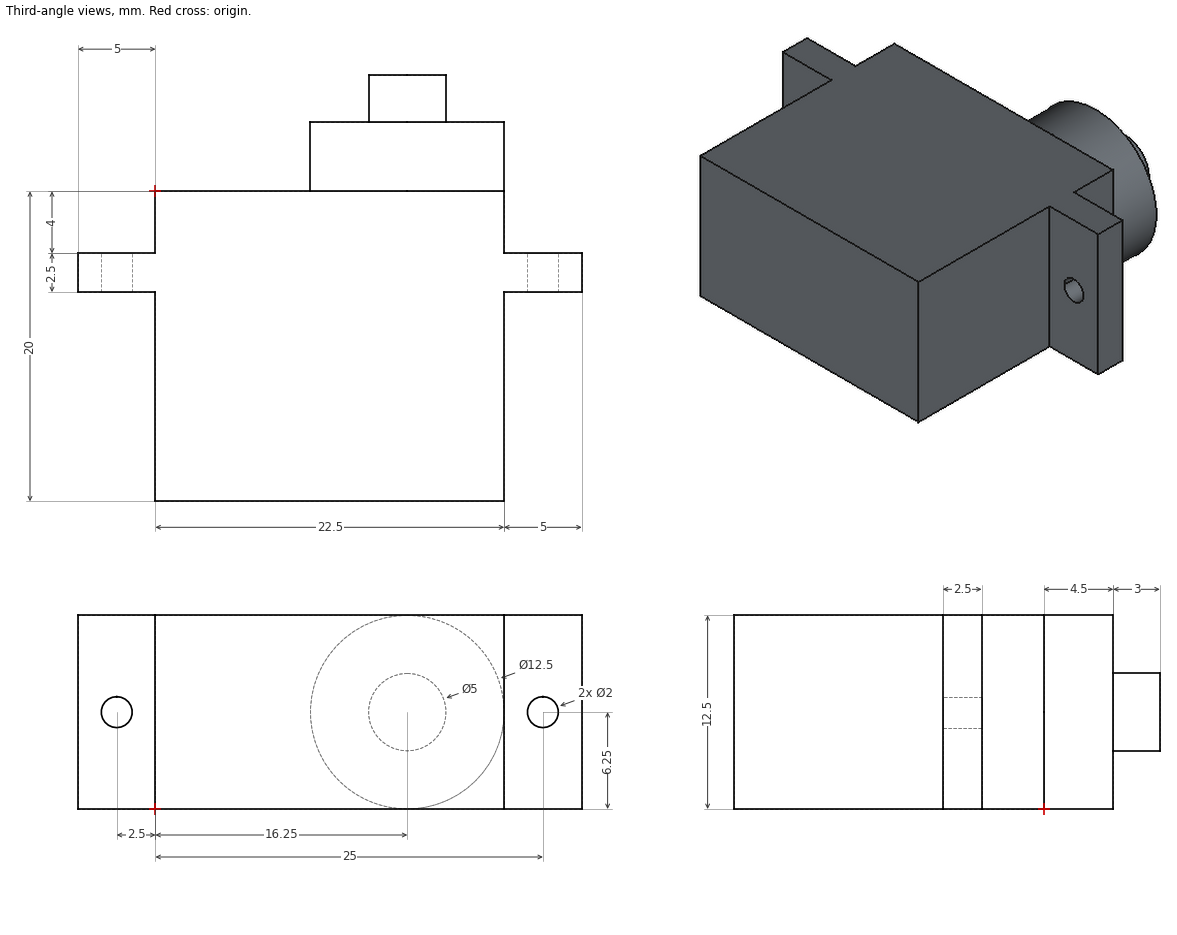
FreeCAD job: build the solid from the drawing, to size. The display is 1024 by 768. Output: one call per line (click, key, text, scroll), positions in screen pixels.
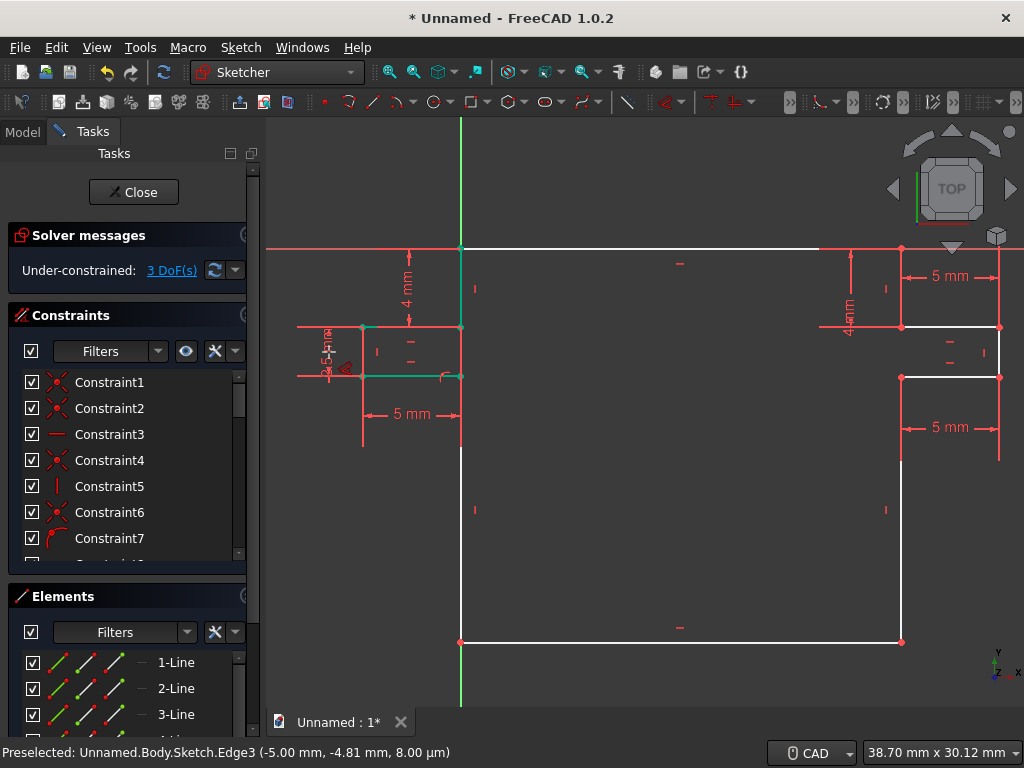
scroll(364, 345, down, 2)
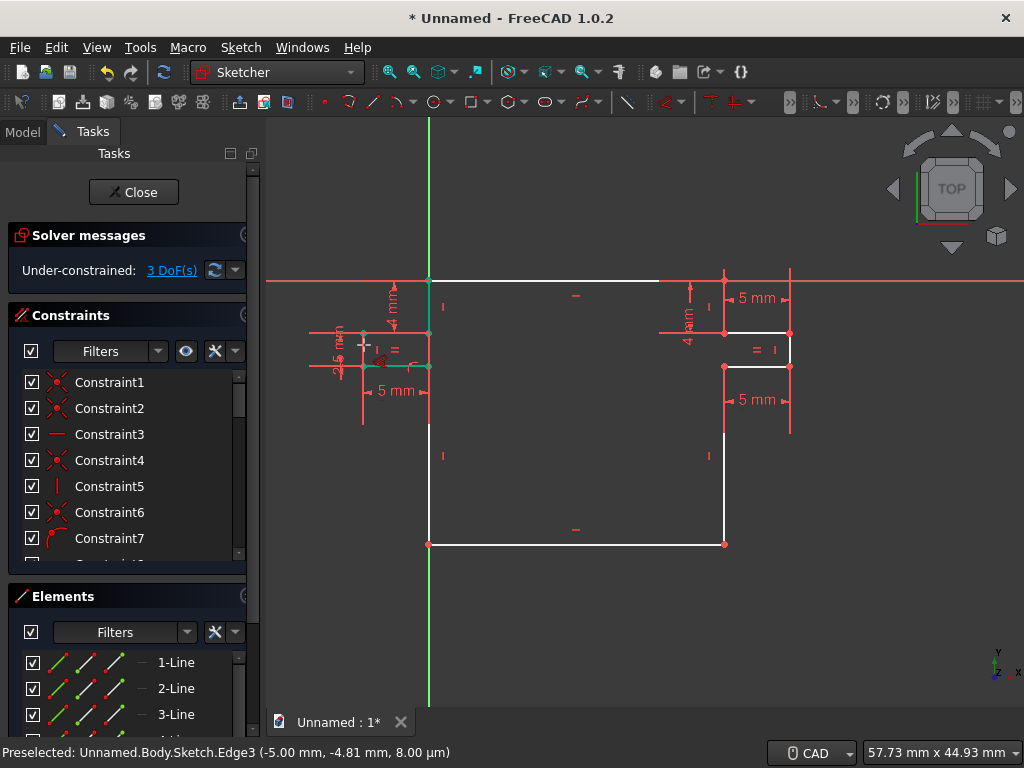
scroll(790, 357, up, 2)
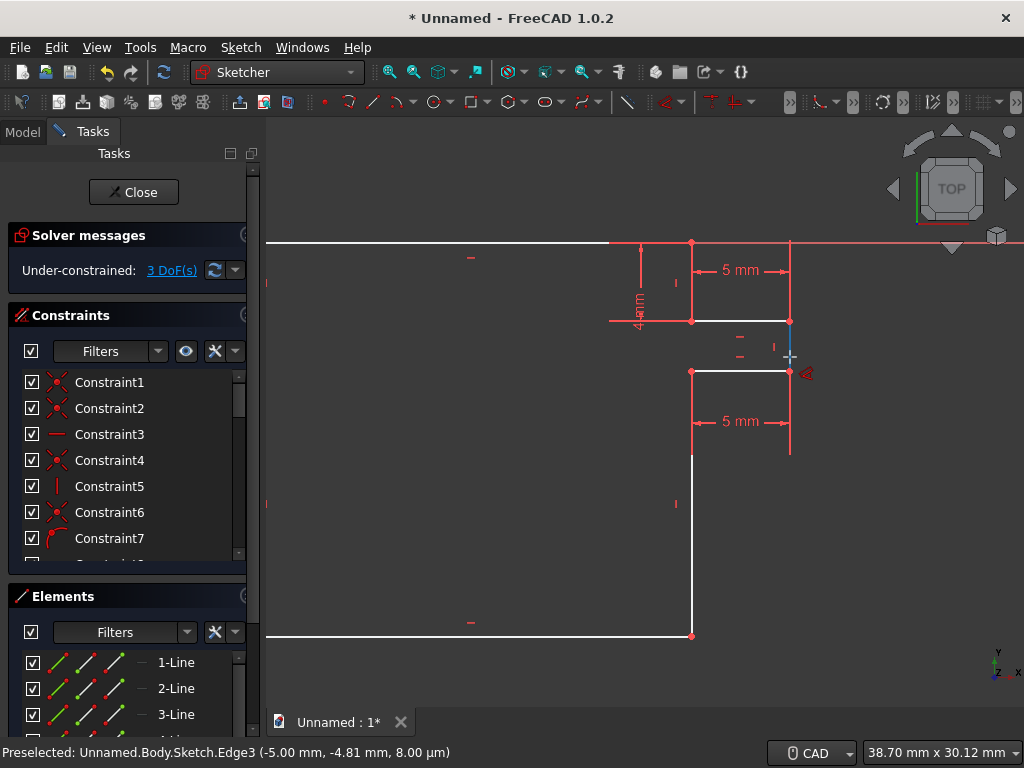
click(790, 356)
click(824, 346)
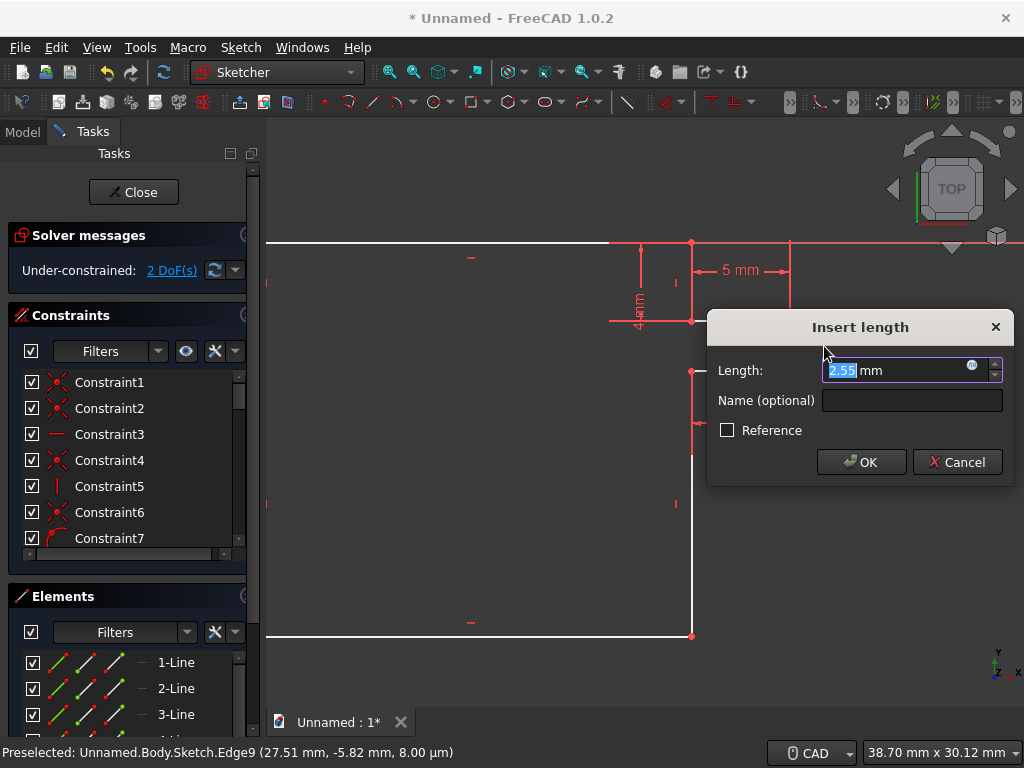
text(2.5)
key(Return)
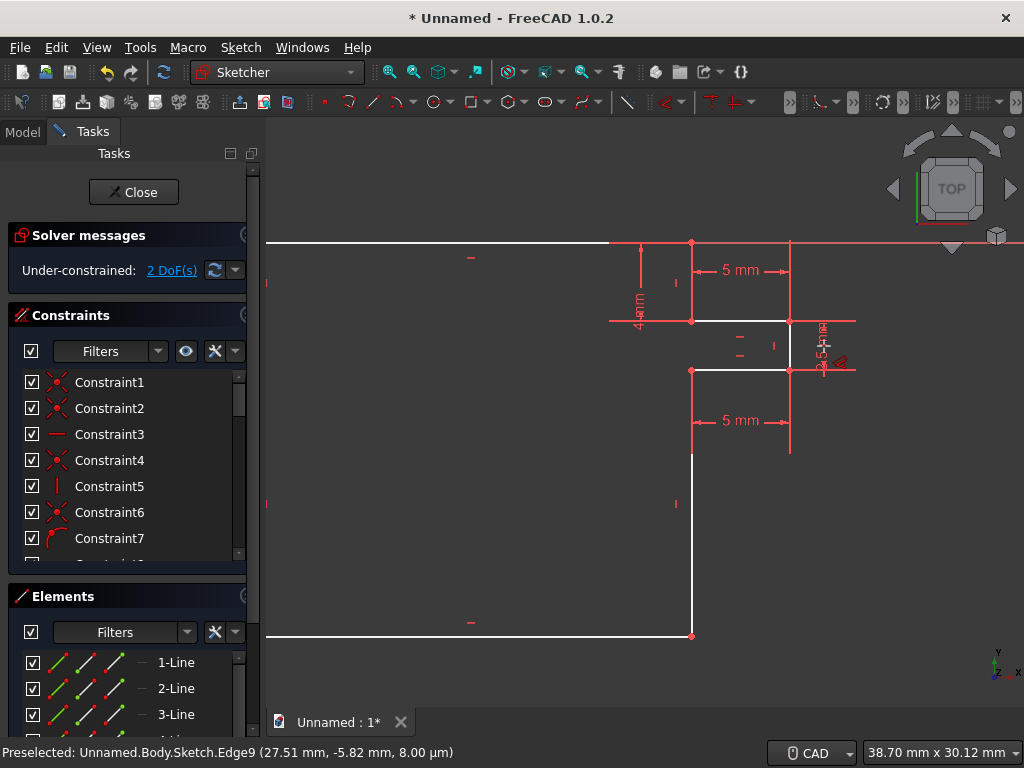
scroll(791, 357, down, 2)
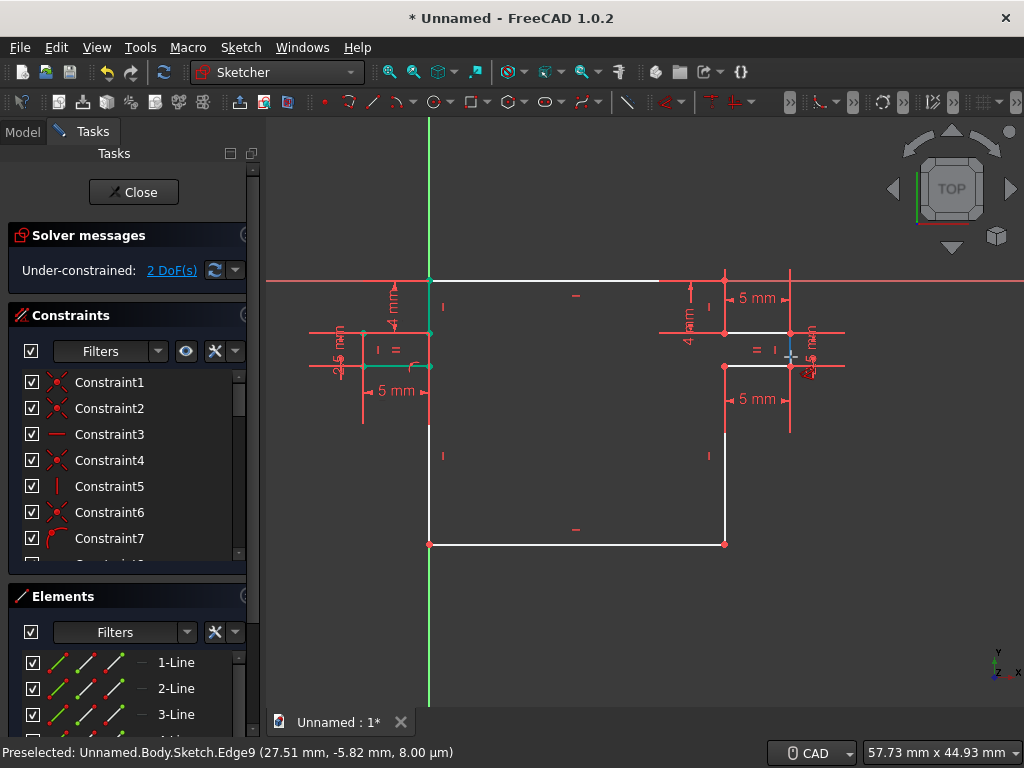
click(429, 545)
click(395, 413)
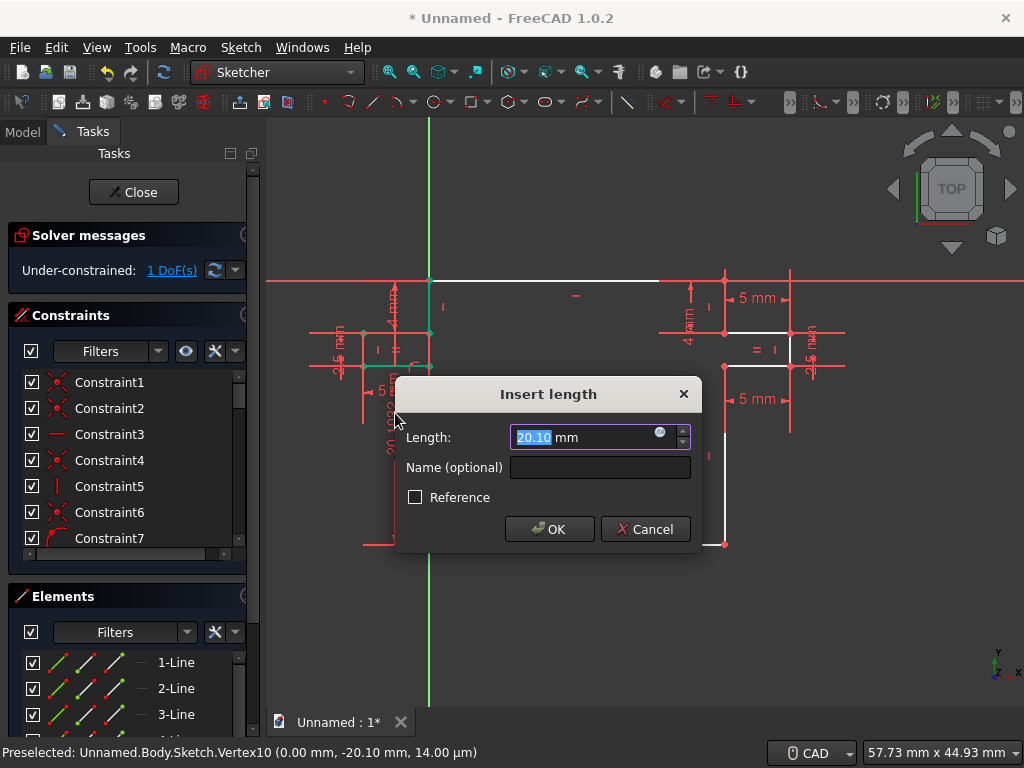
text(20)
key(Return)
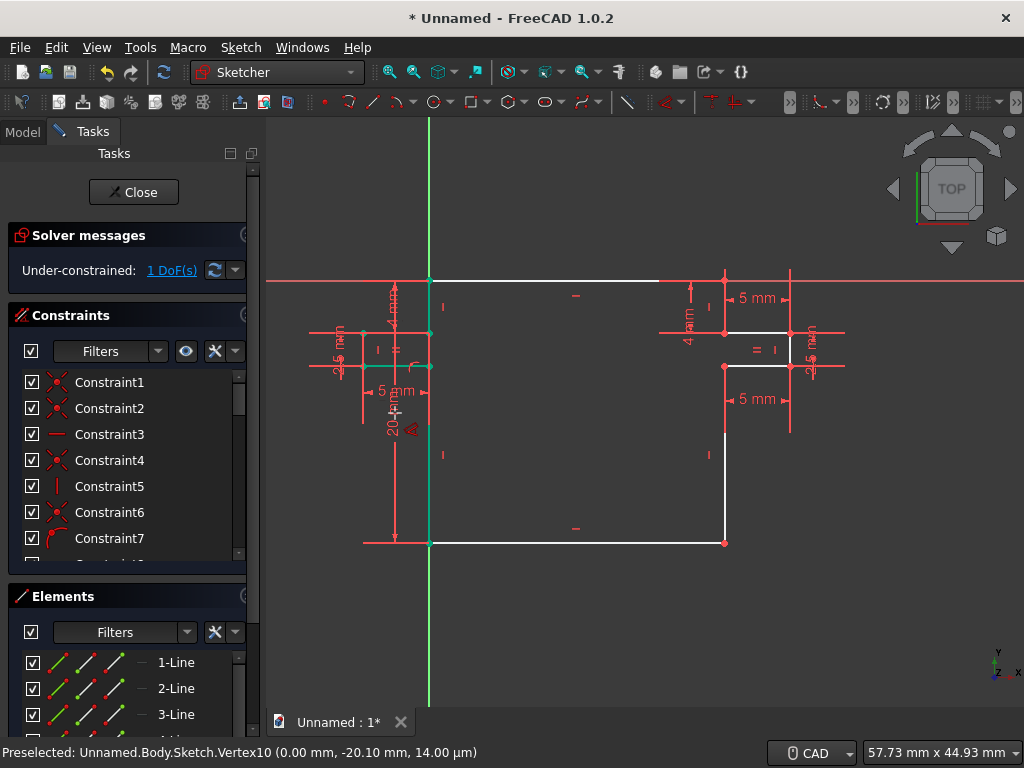
click(518, 543)
click(577, 577)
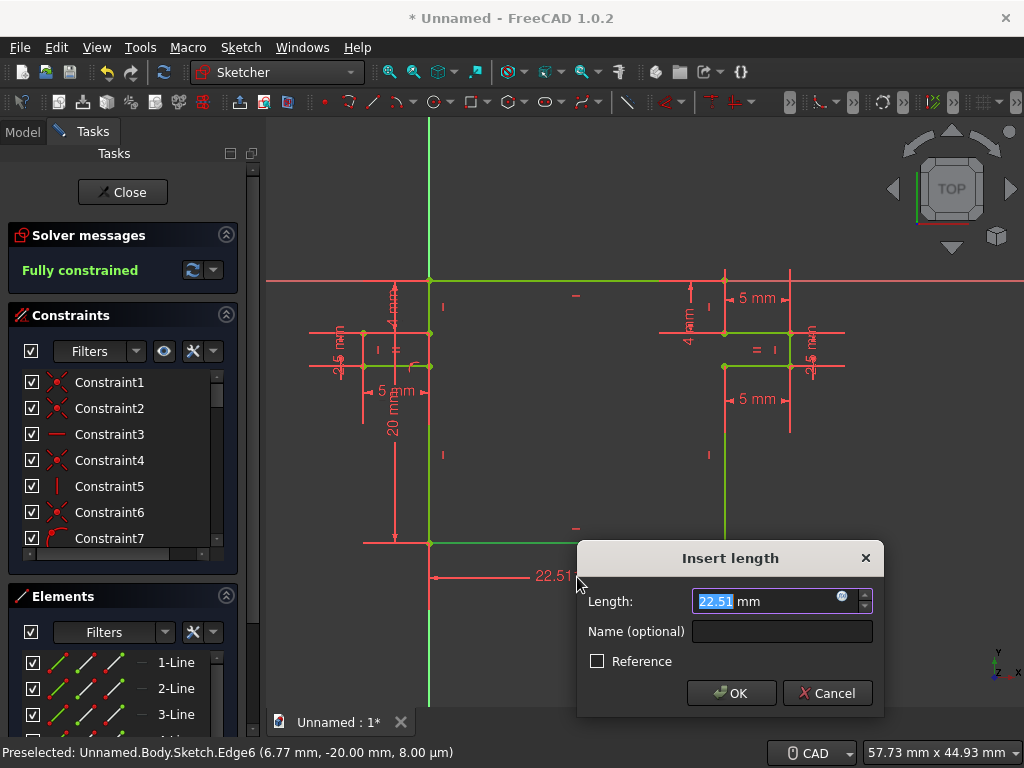
text(22.5)
key(Return)
key(Escape)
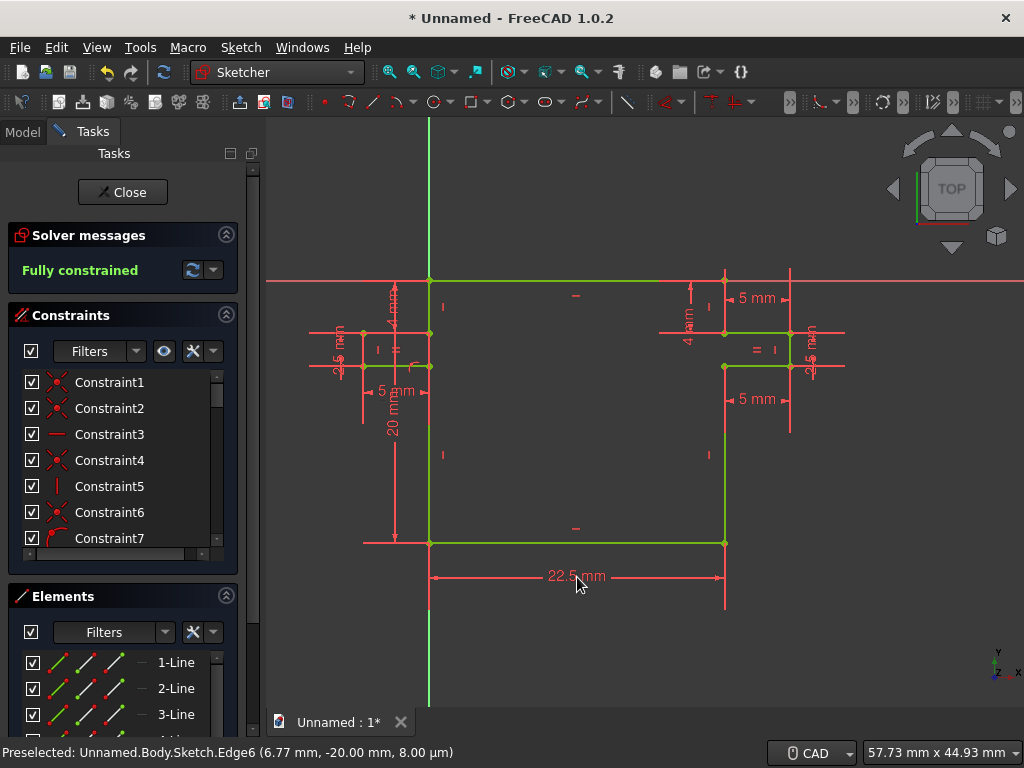
click(123, 192)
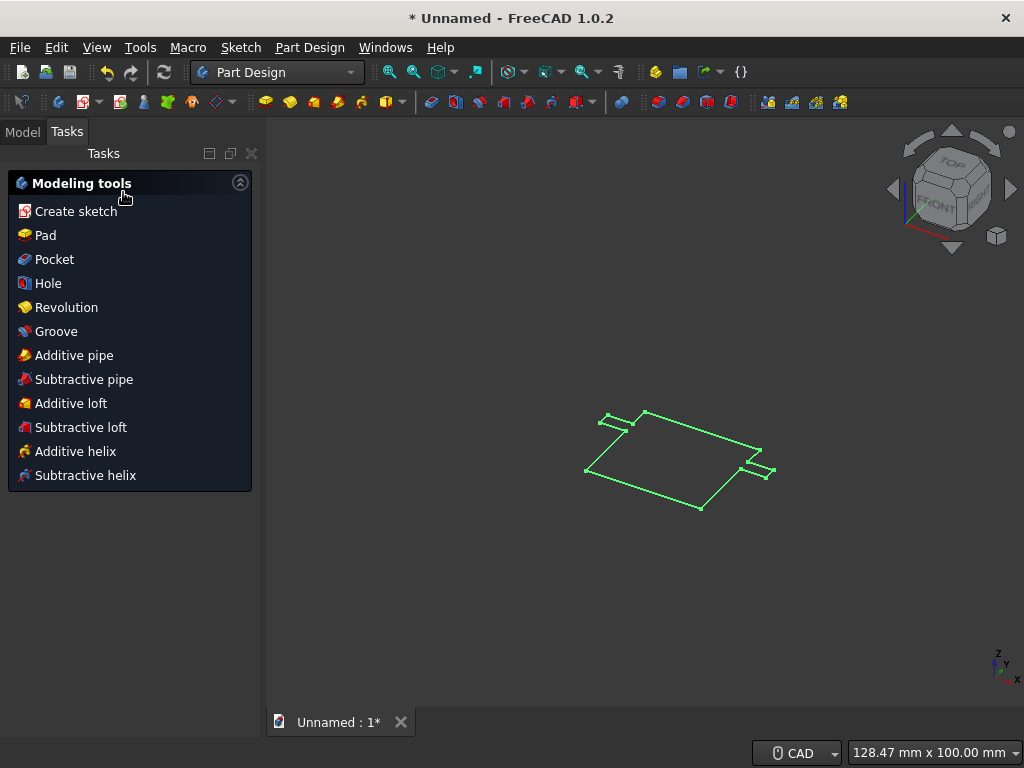
click(266, 102)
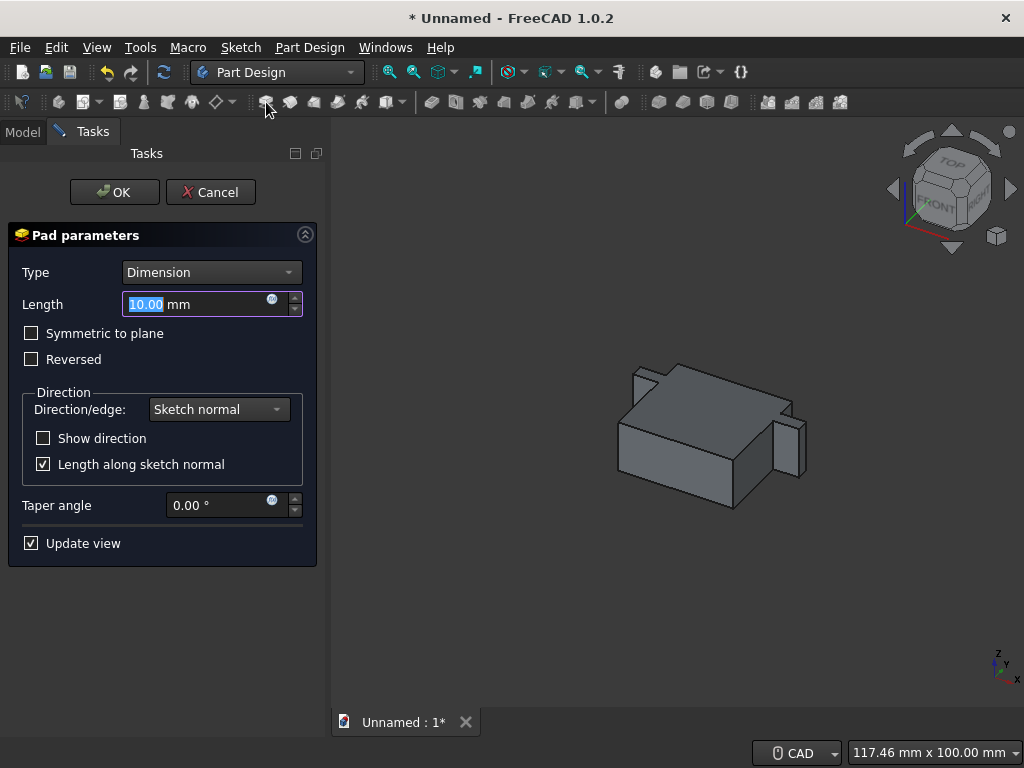
text(12.5)
key(Tab)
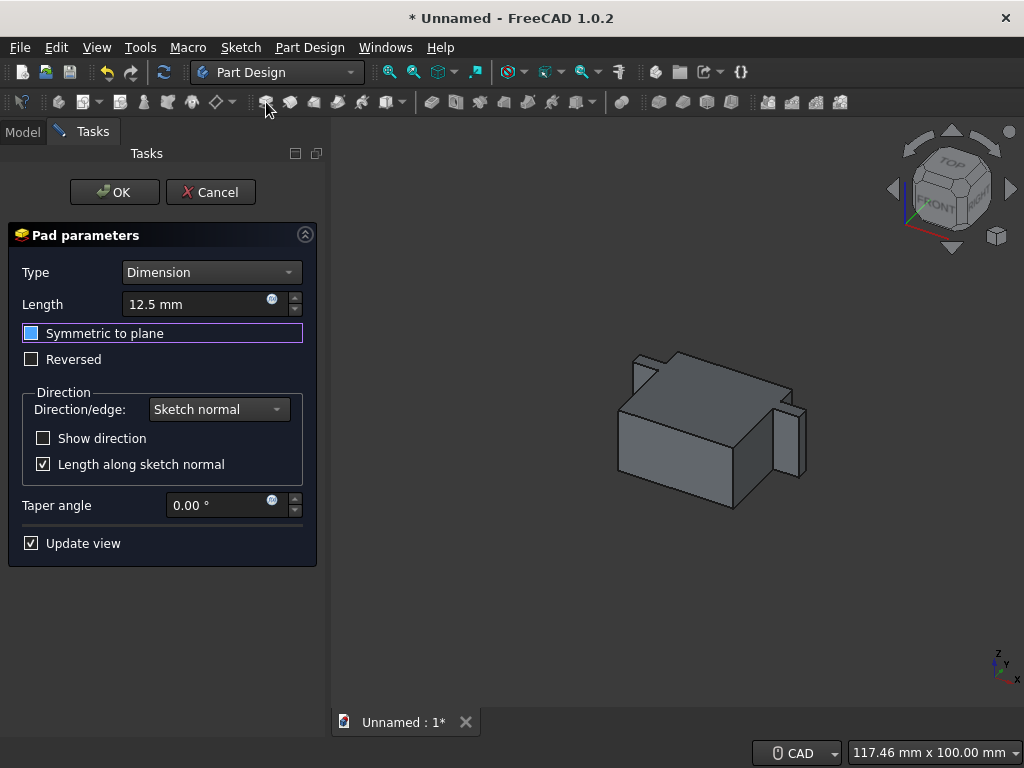
click(115, 192)